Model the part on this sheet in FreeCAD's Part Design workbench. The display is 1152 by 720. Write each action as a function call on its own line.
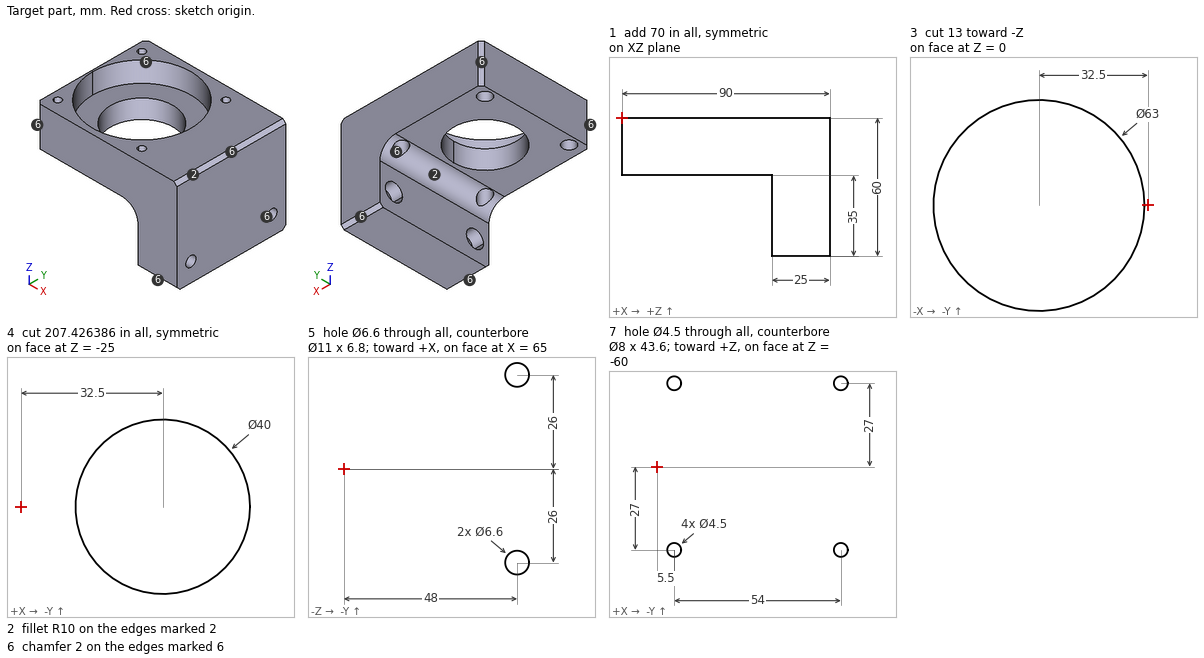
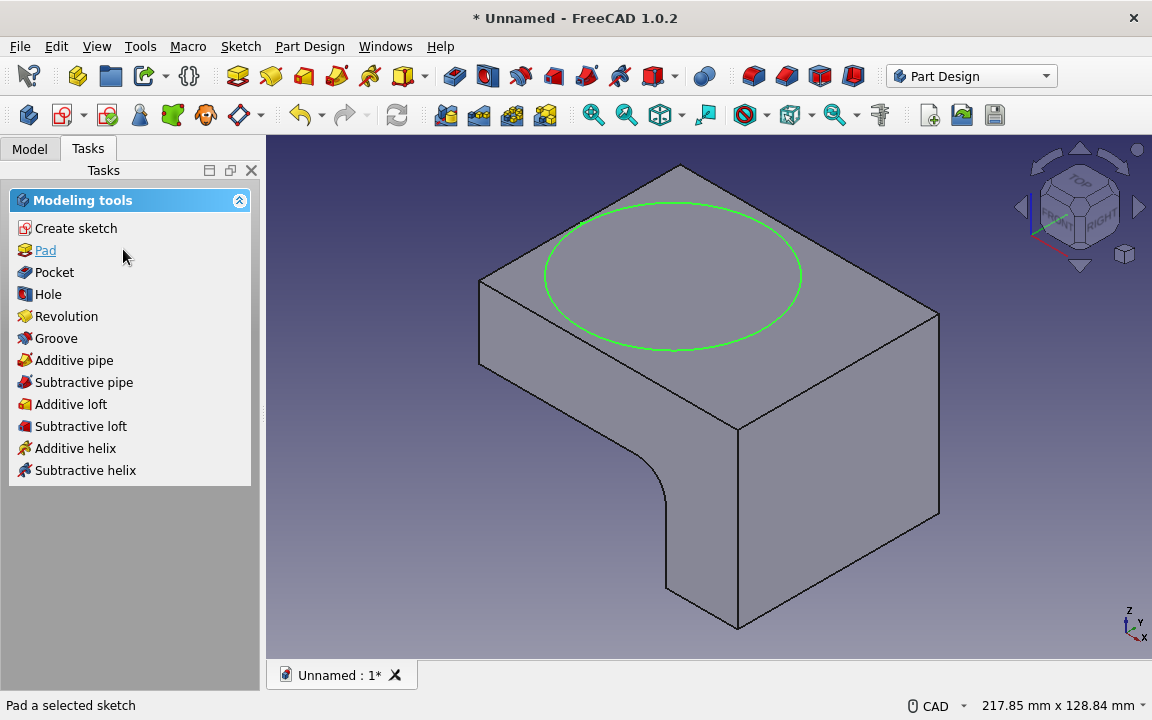
click(455, 76)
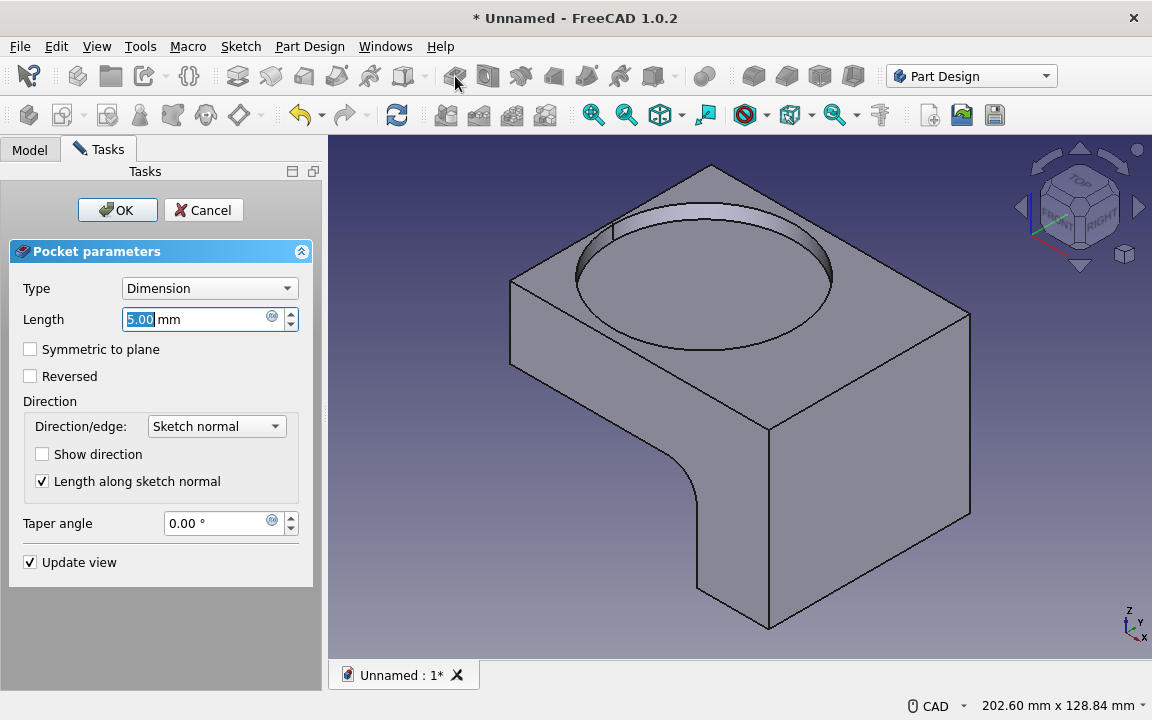
text(13)
key(Tab)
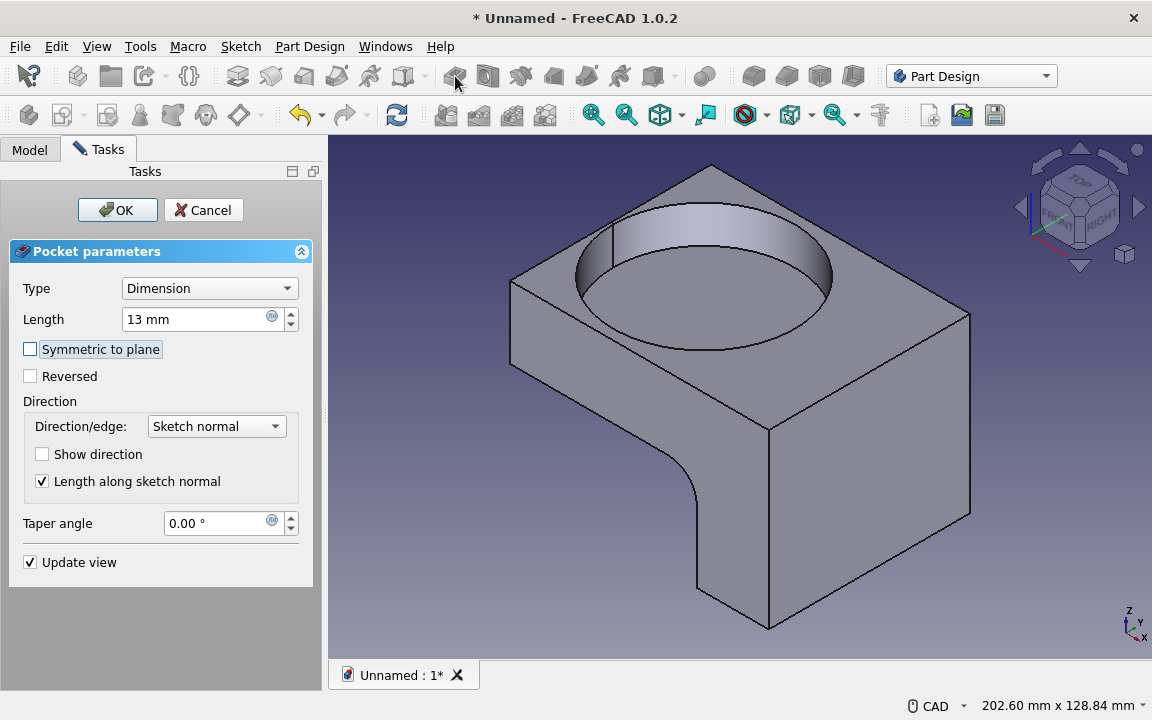
click(118, 210)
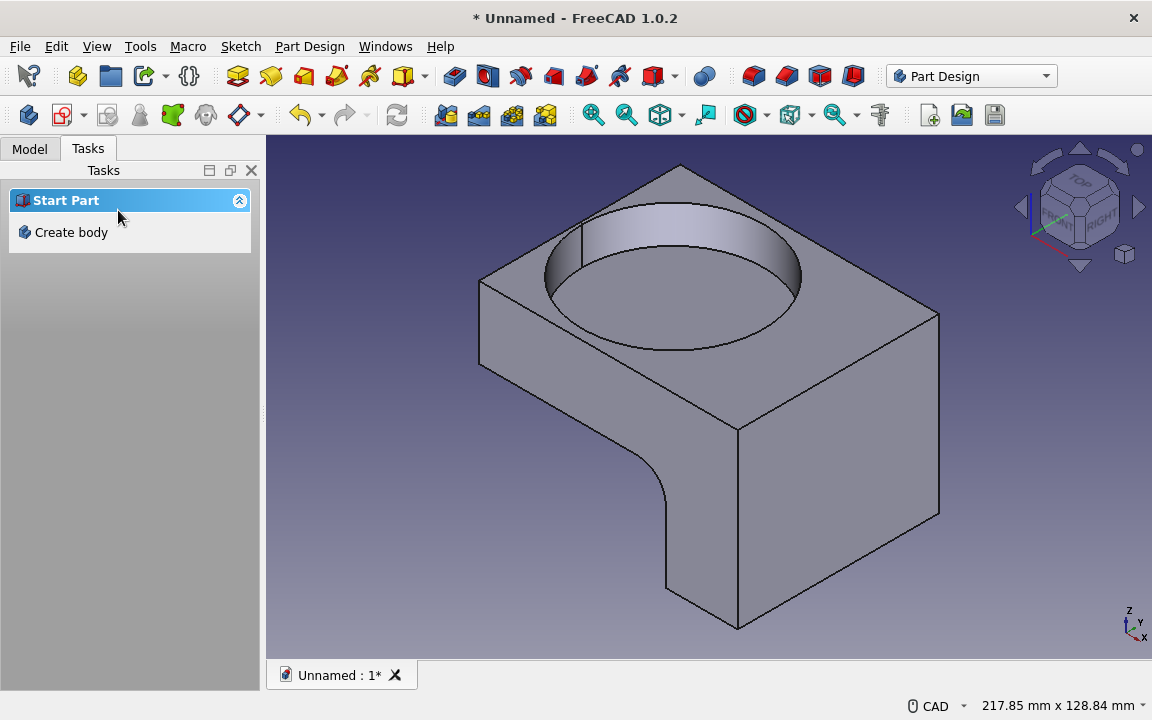
key(5)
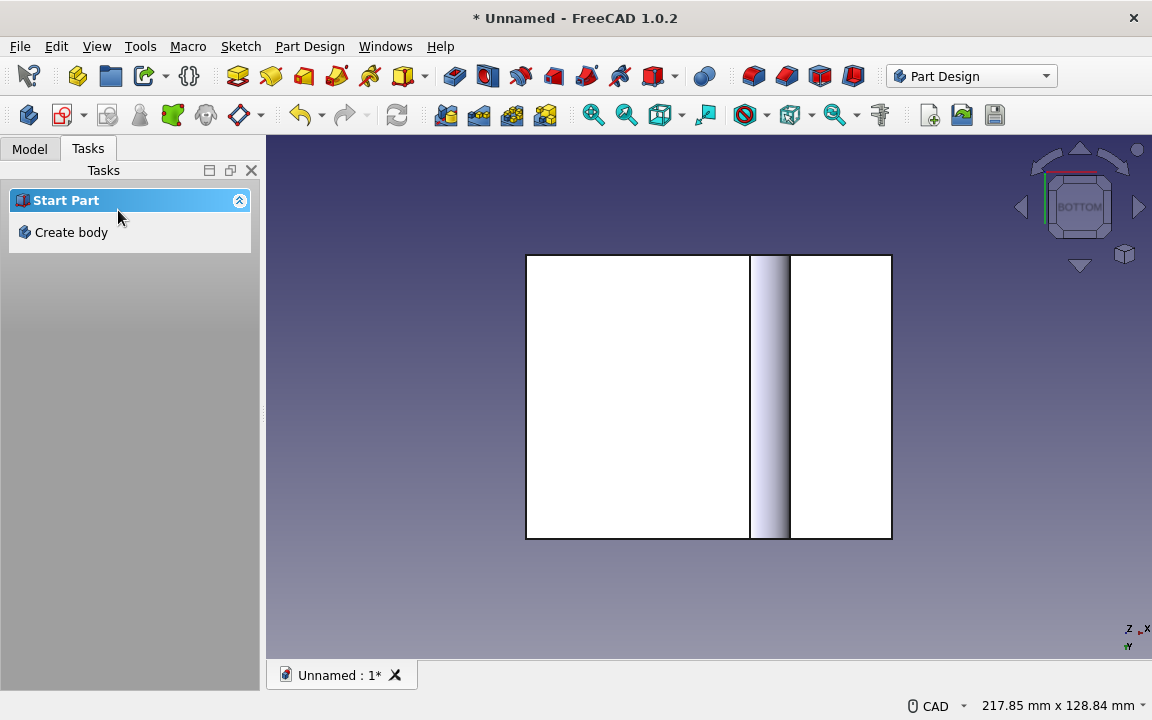
click(638, 396)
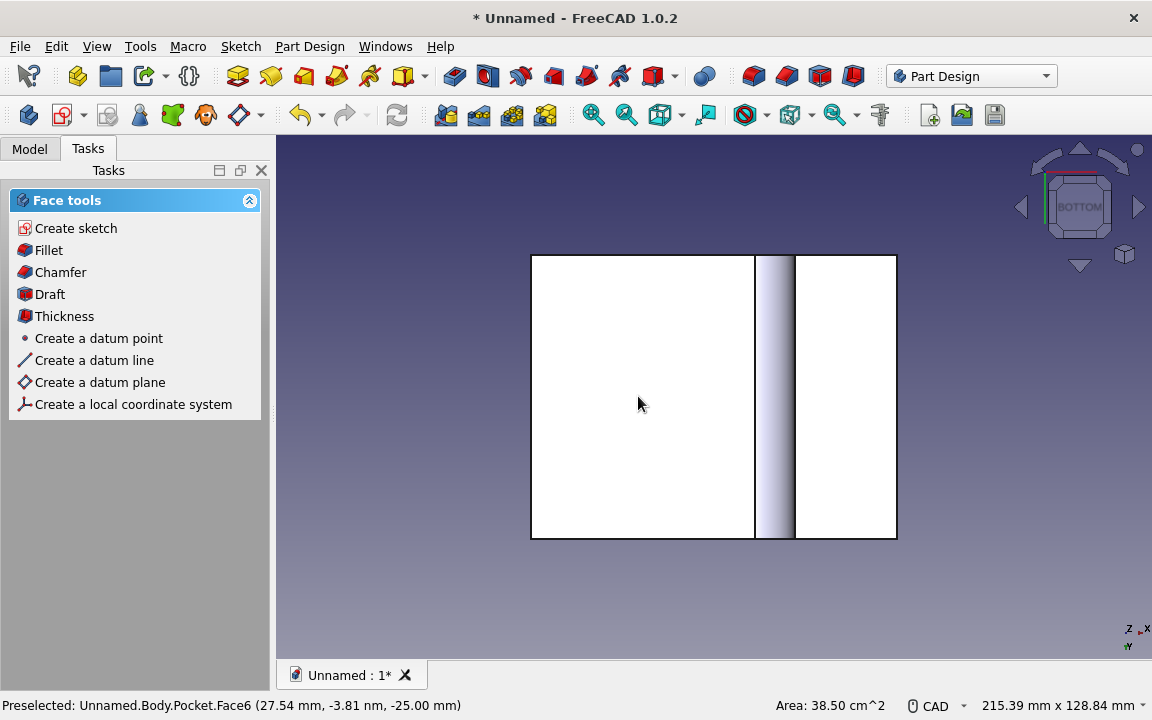
click(62, 116)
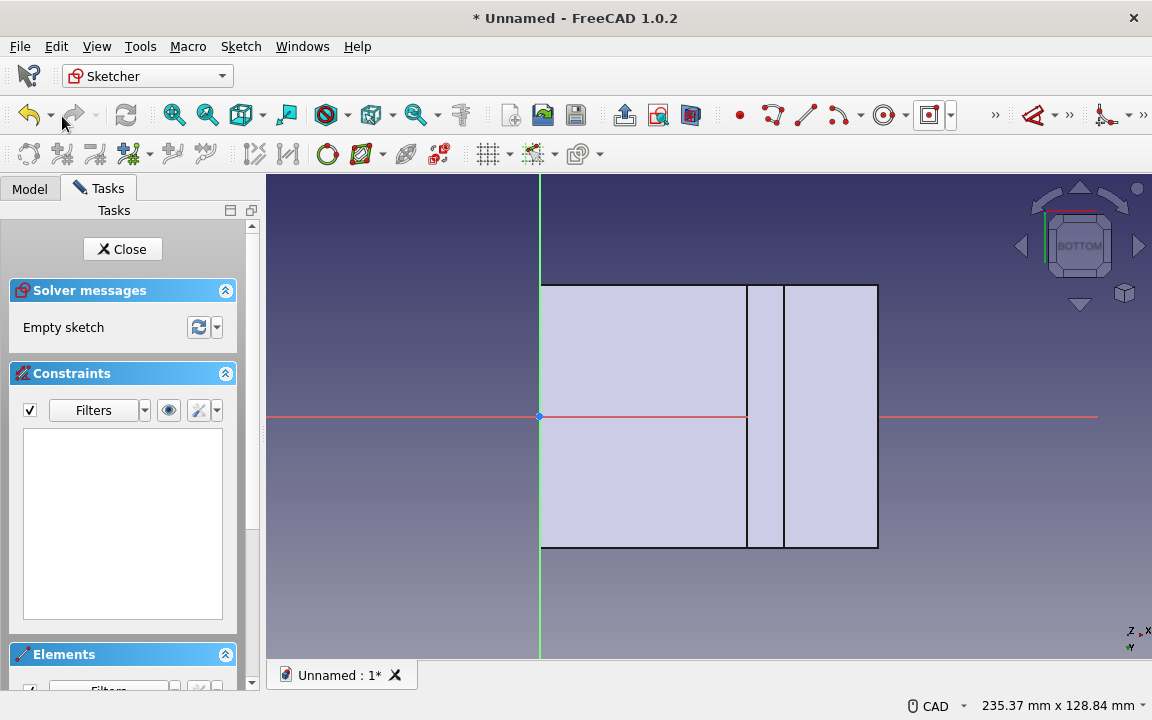
key(q)
key(s)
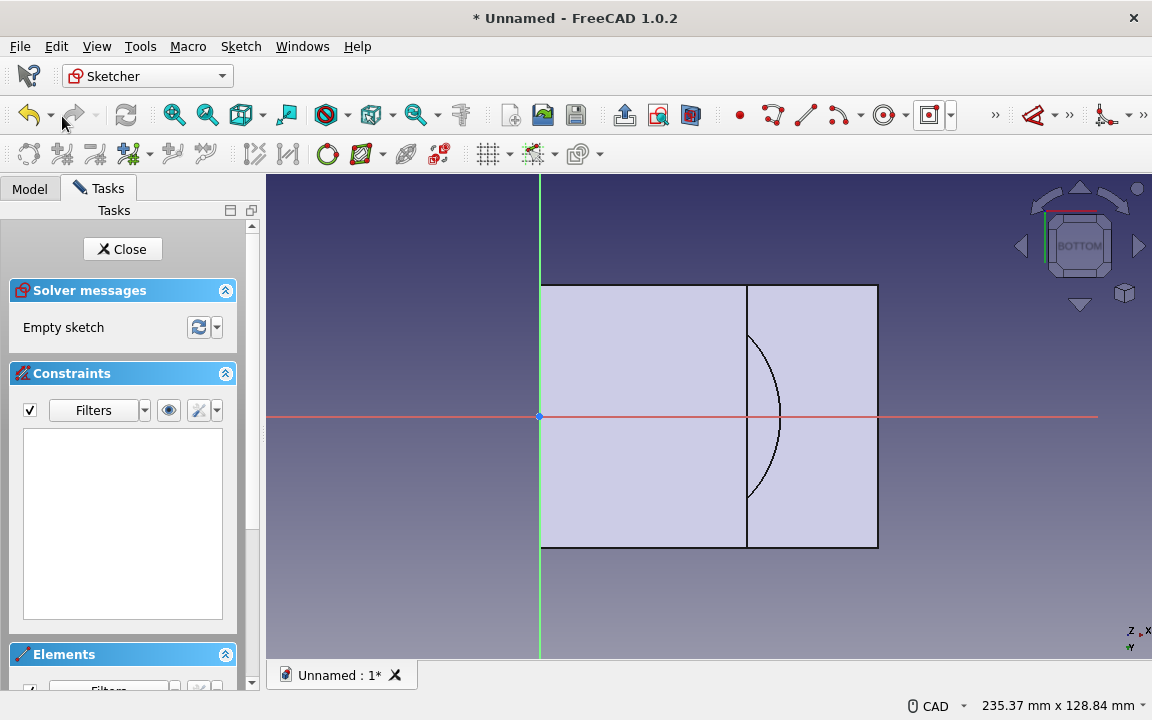
scroll(636, 417, up, 3)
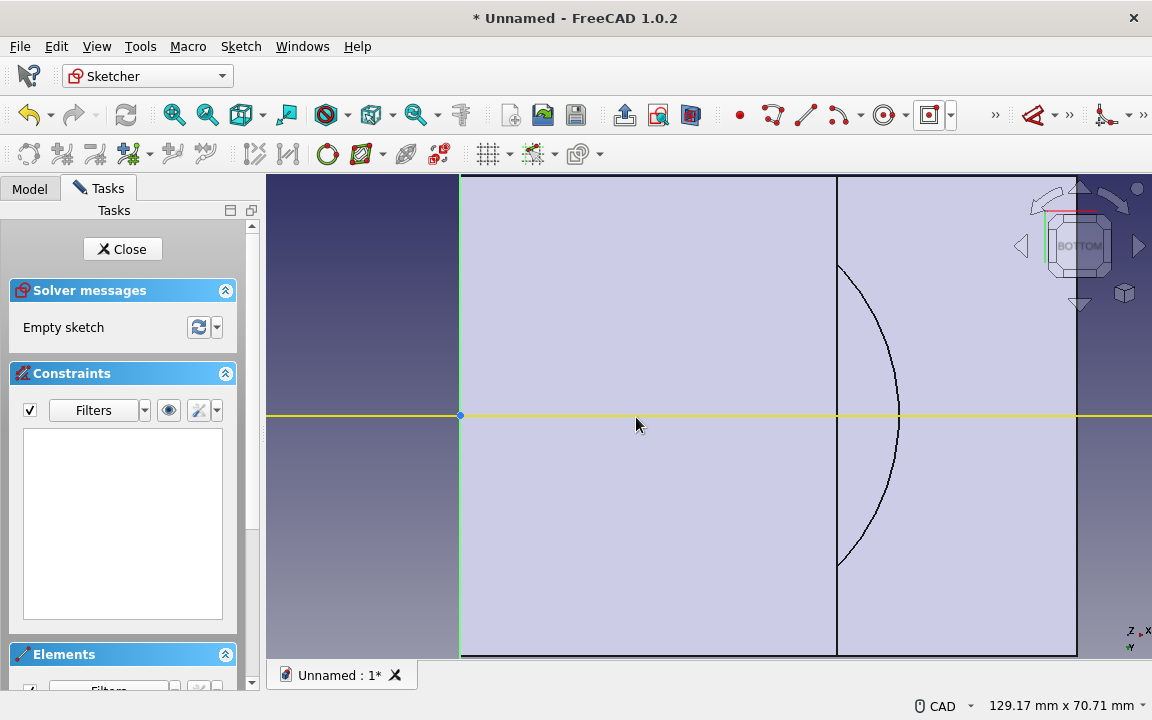
click(884, 116)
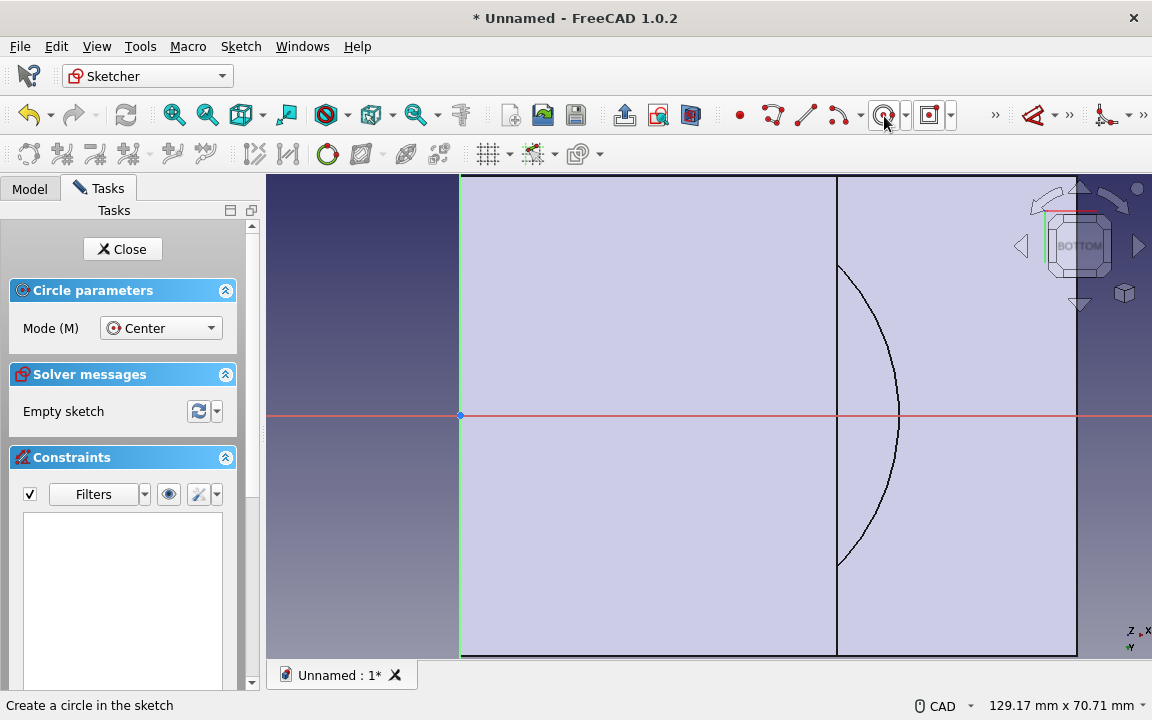
click(683, 416)
move(780, 319)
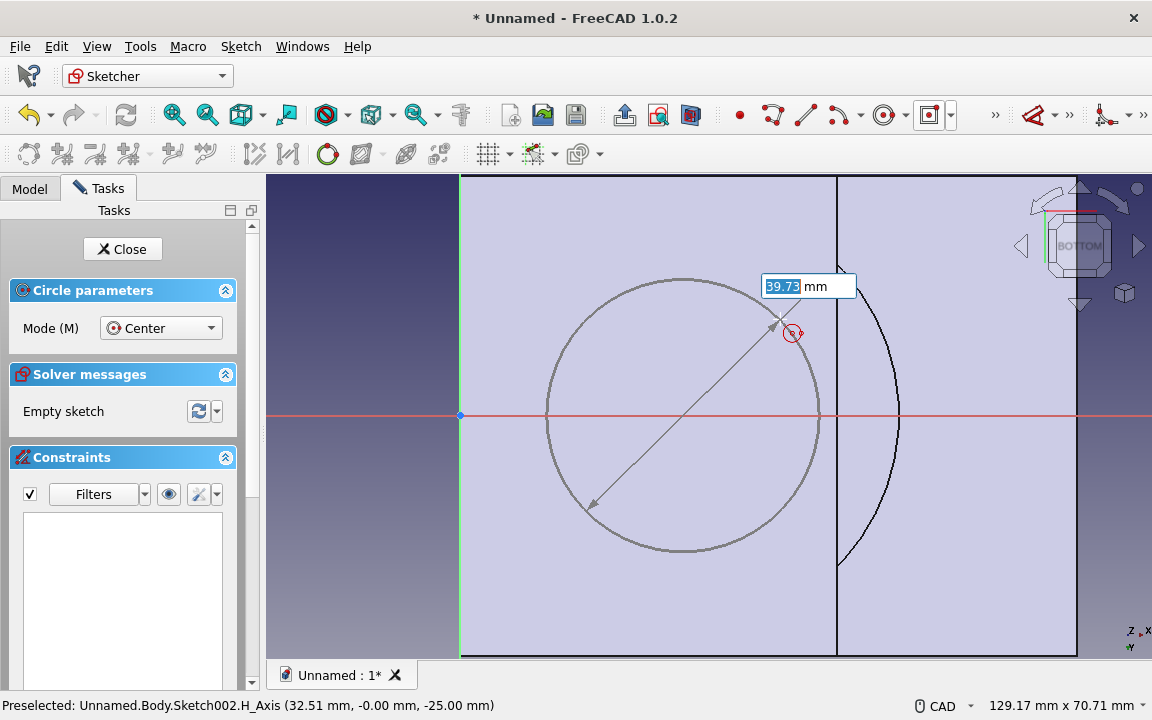
text(40)
key(Return)
key(Escape)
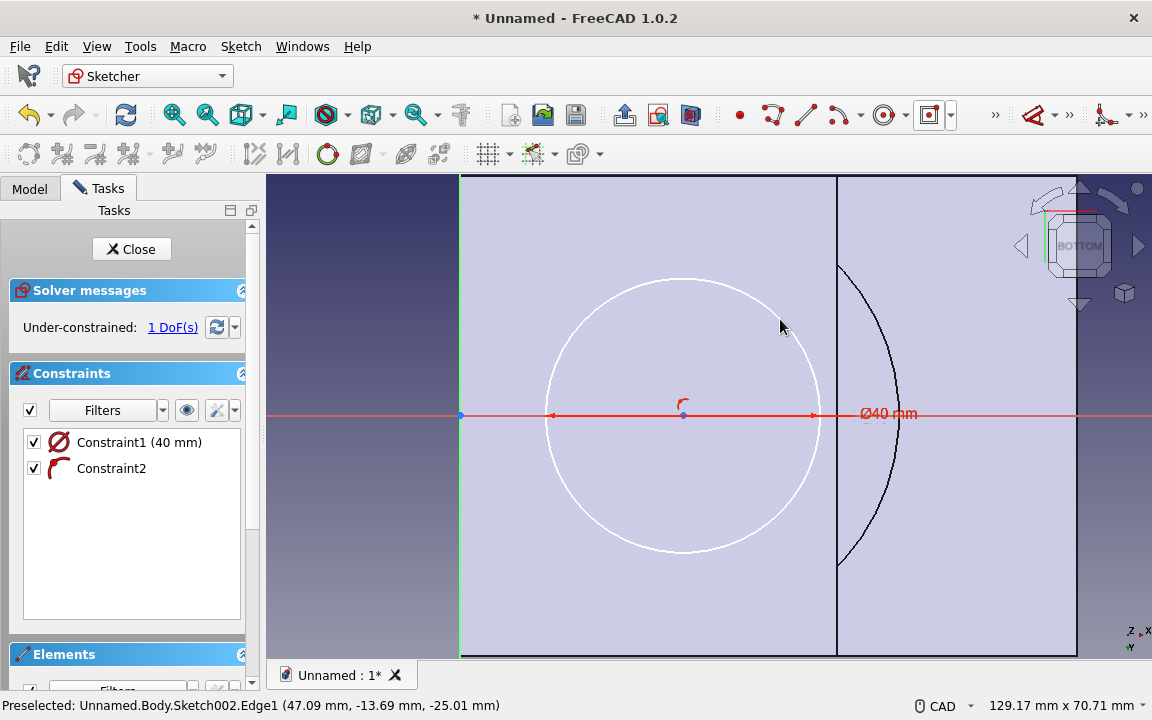
key(d)